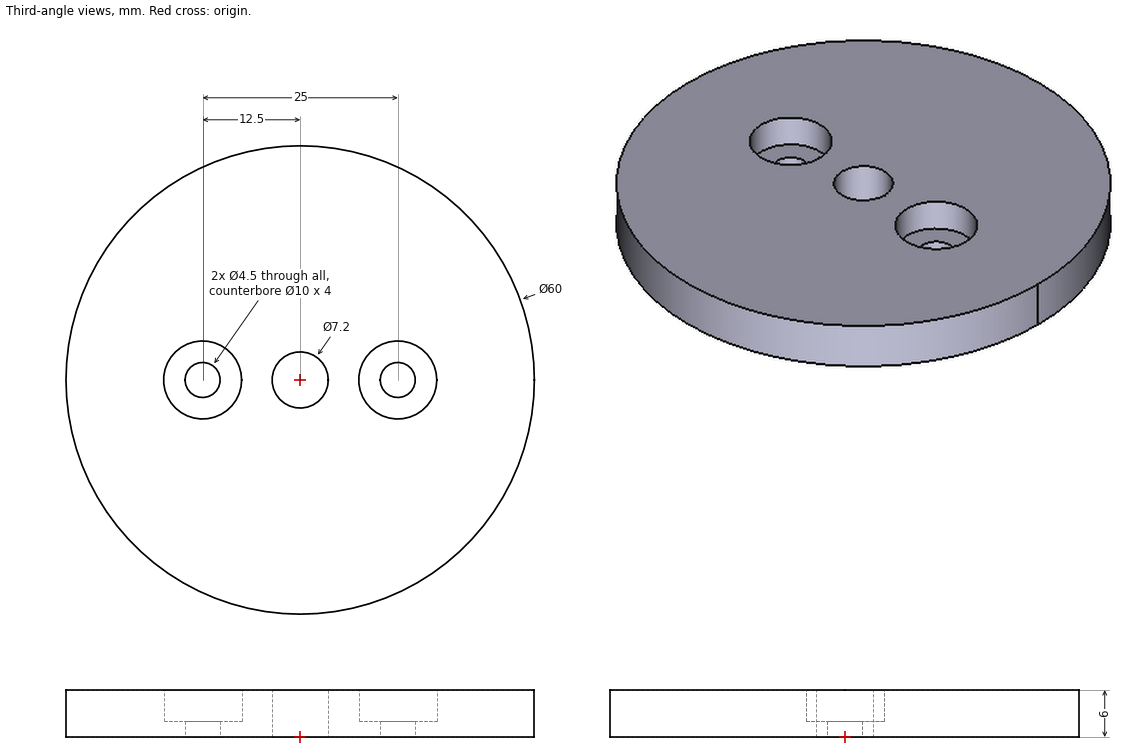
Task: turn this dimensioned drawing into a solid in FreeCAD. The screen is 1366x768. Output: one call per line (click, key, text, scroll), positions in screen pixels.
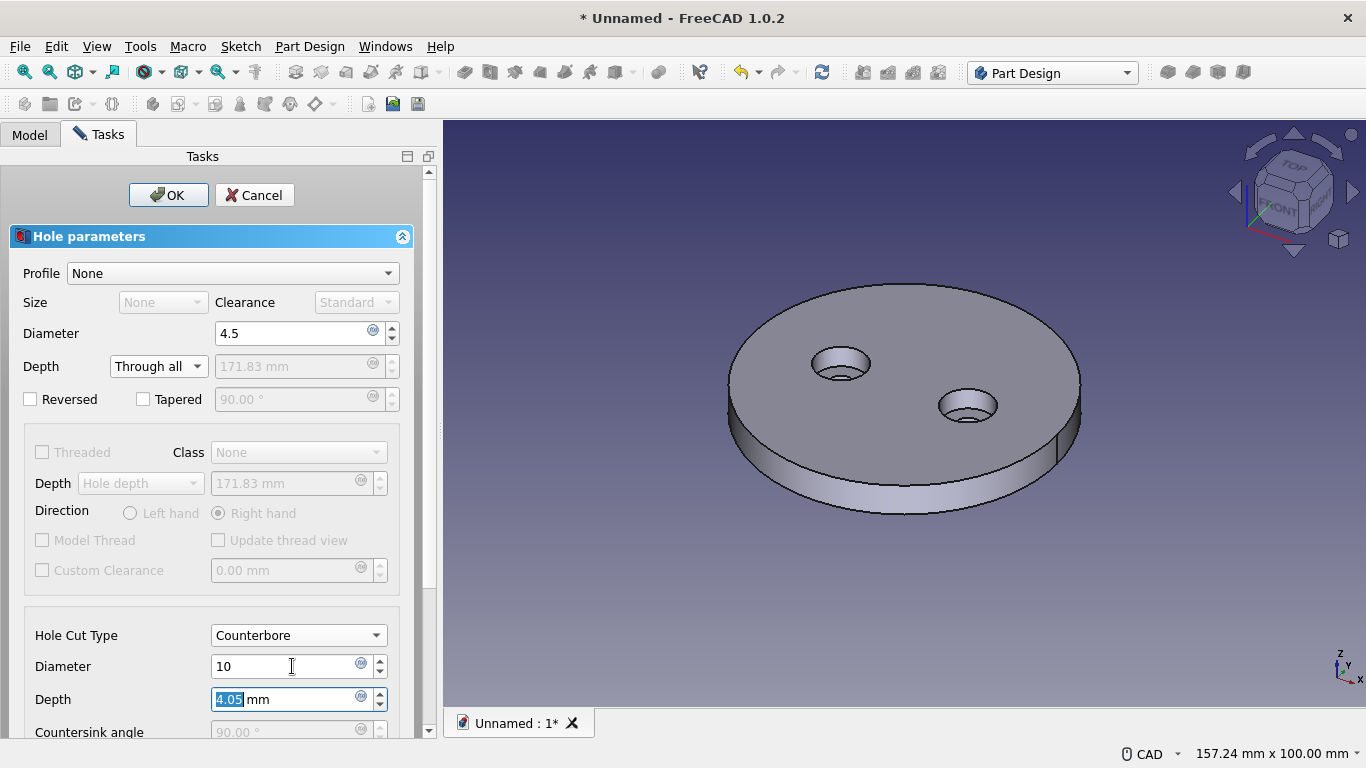
text(4)
key(Tab)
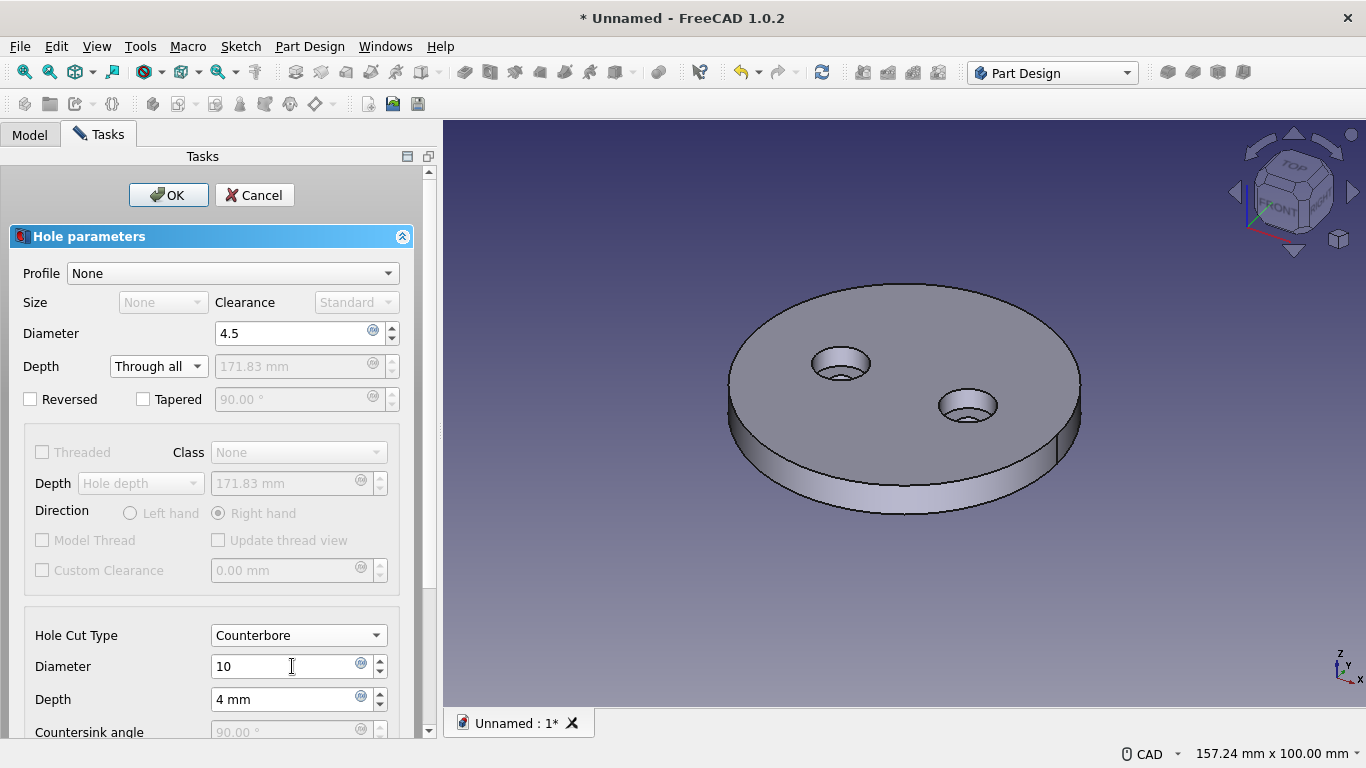
click(169, 195)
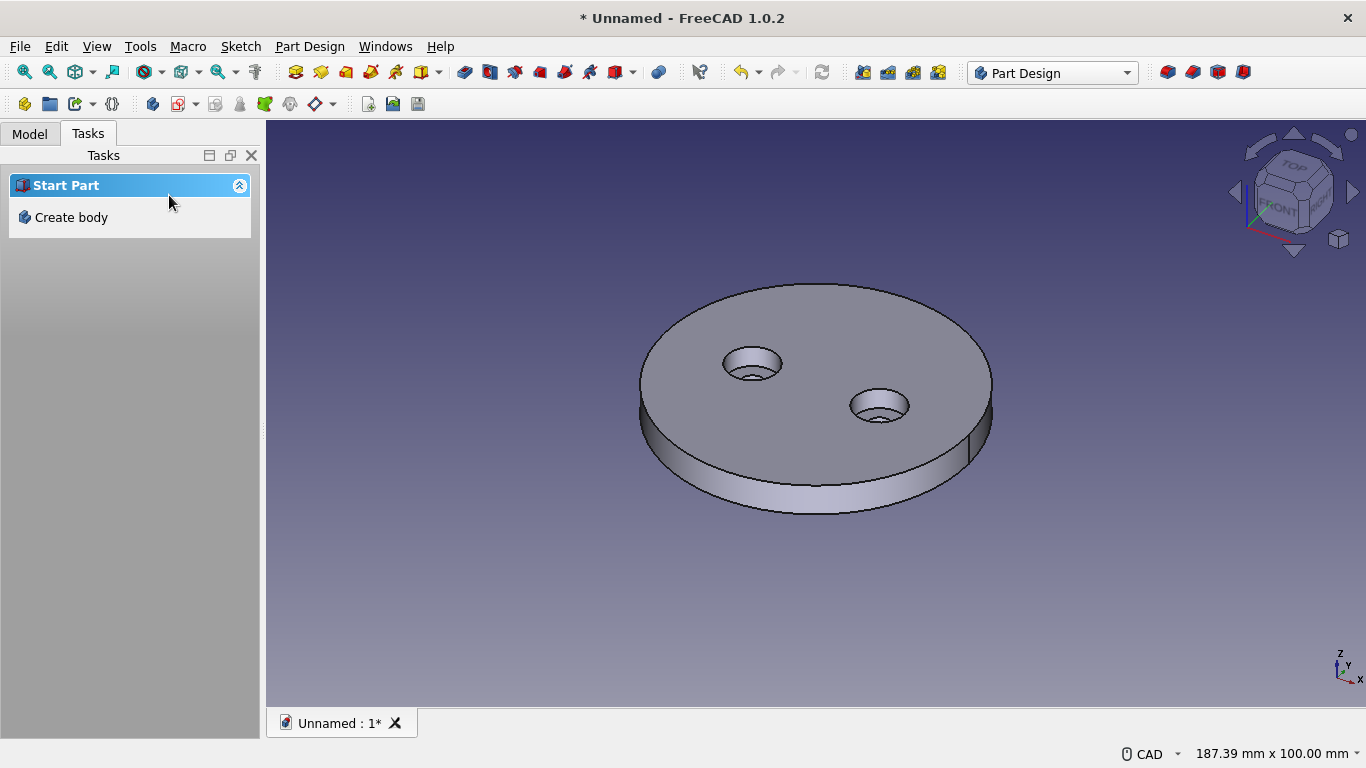
click(766, 434)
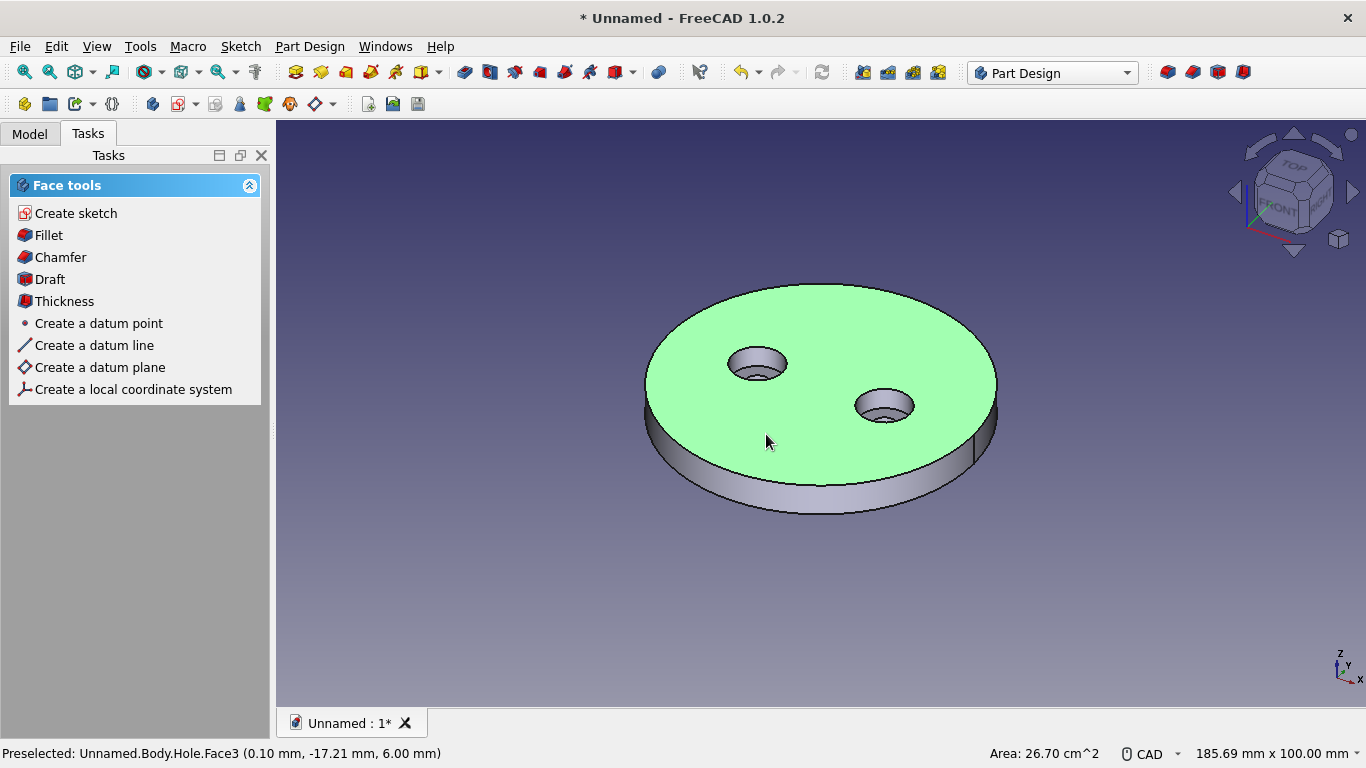
click(178, 104)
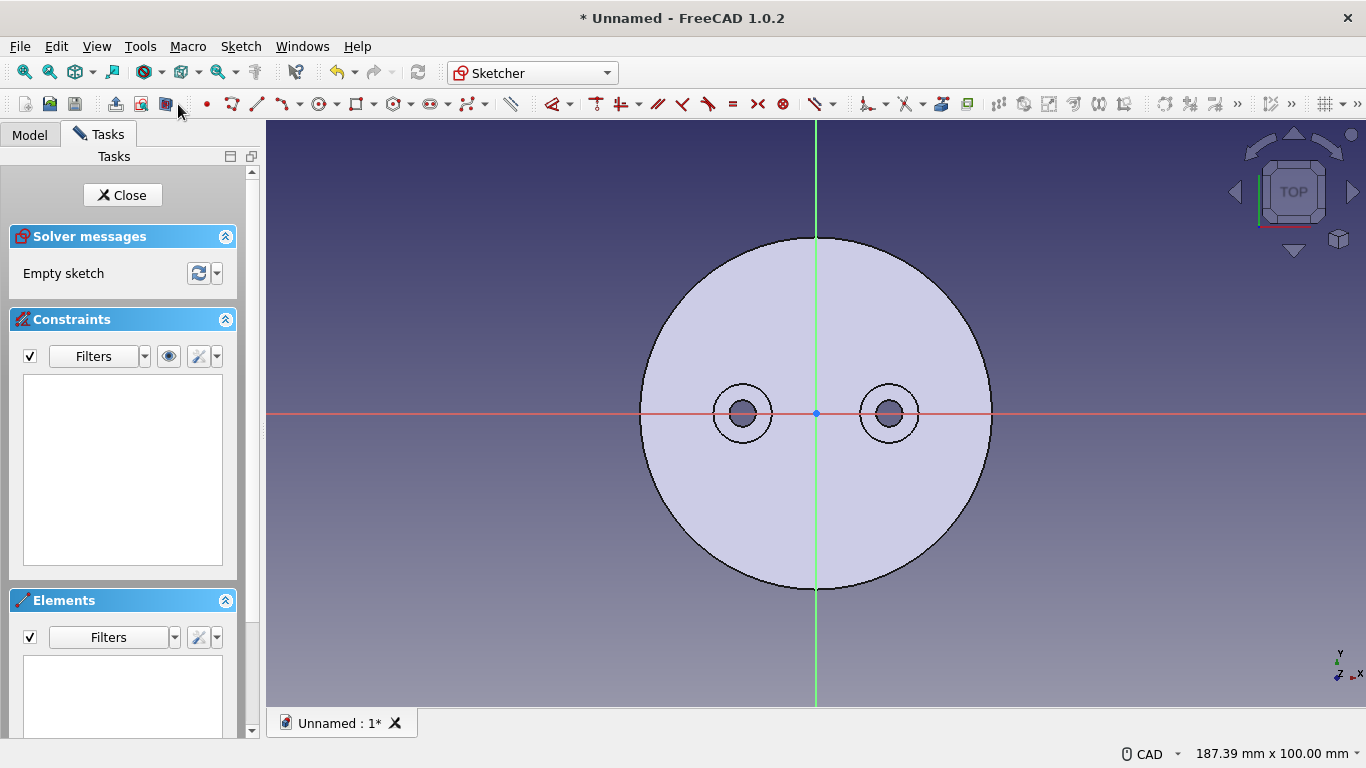
scroll(825, 414, up, 11)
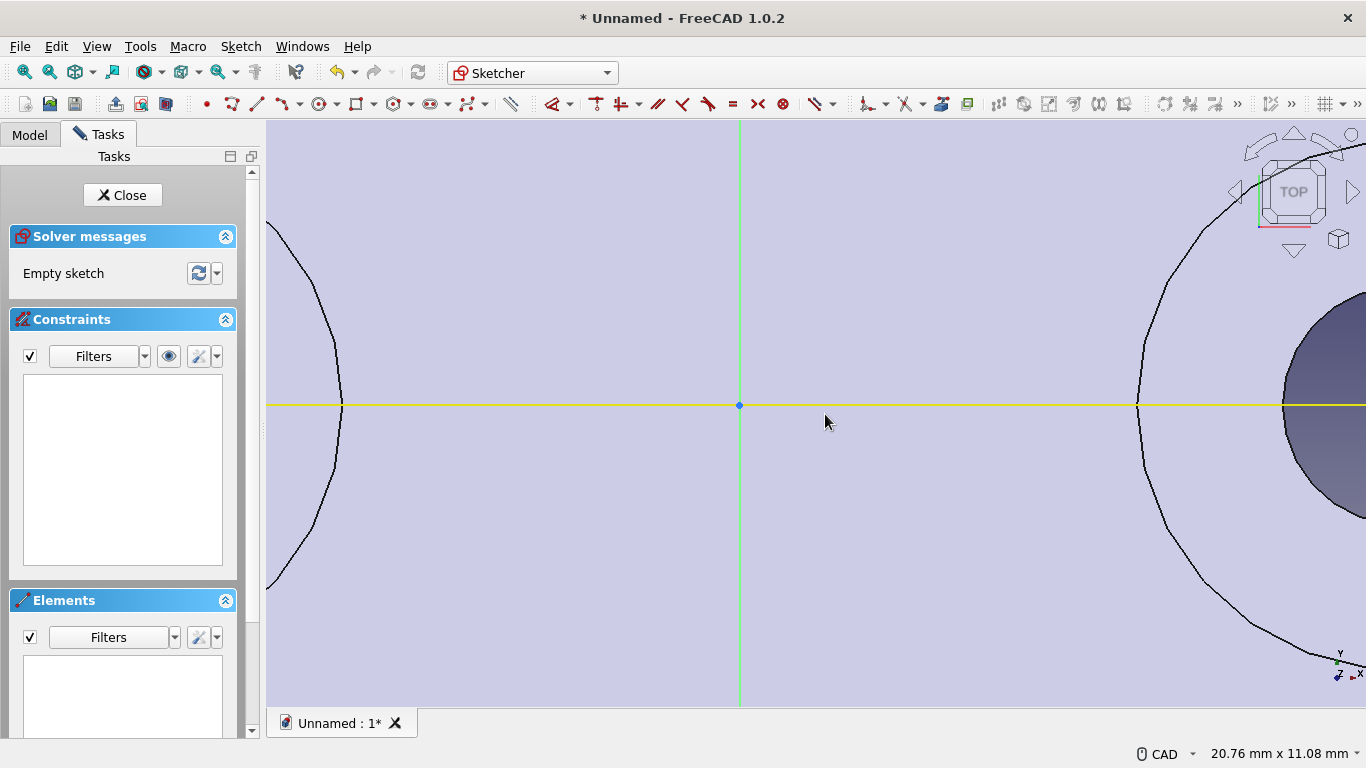
click(318, 104)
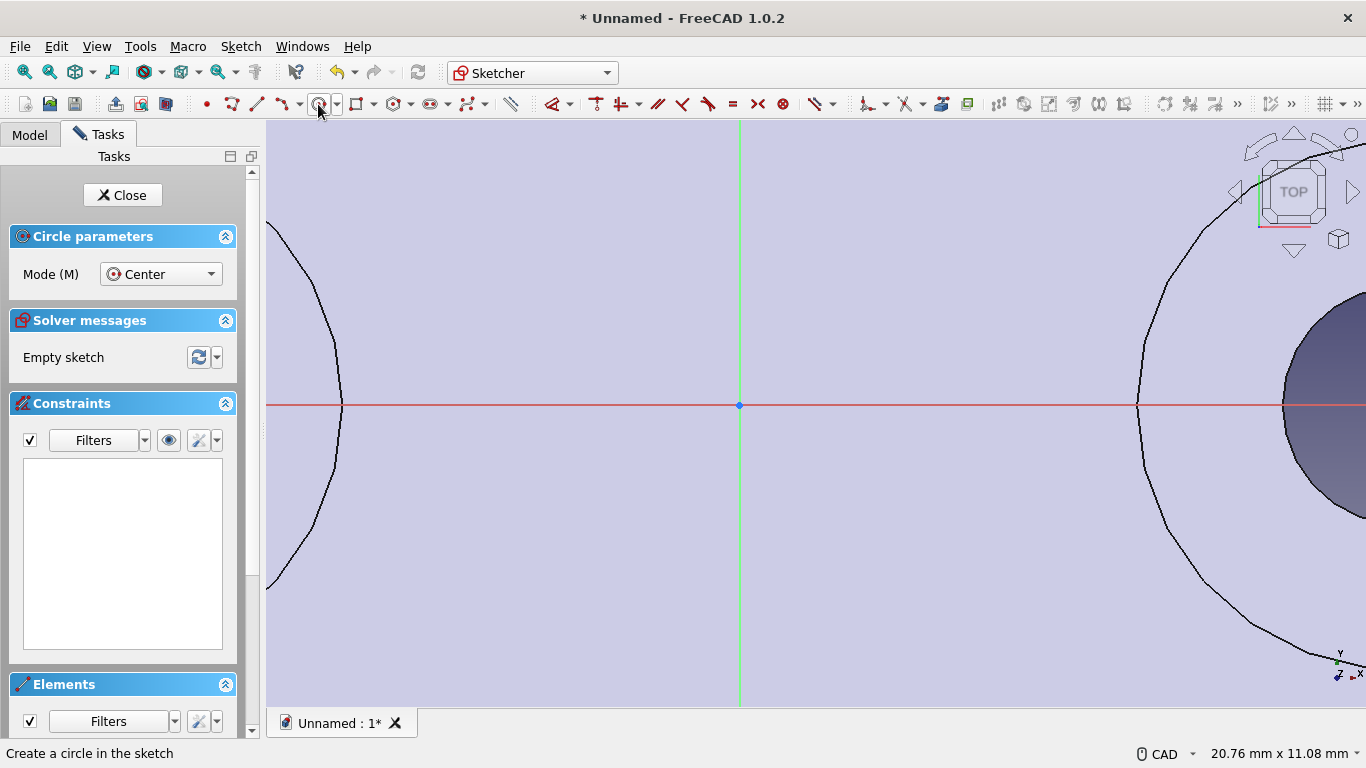
click(740, 405)
click(875, 271)
key(Escape)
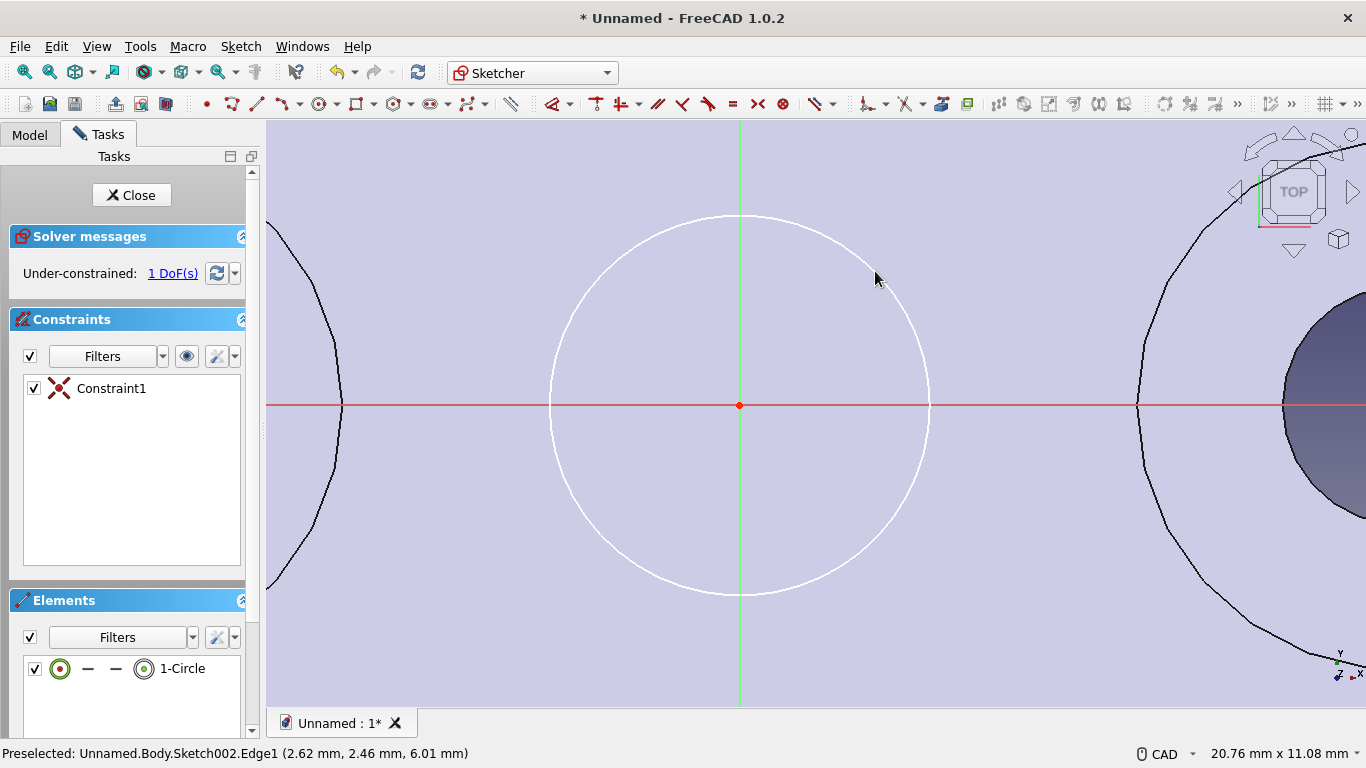
click(552, 104)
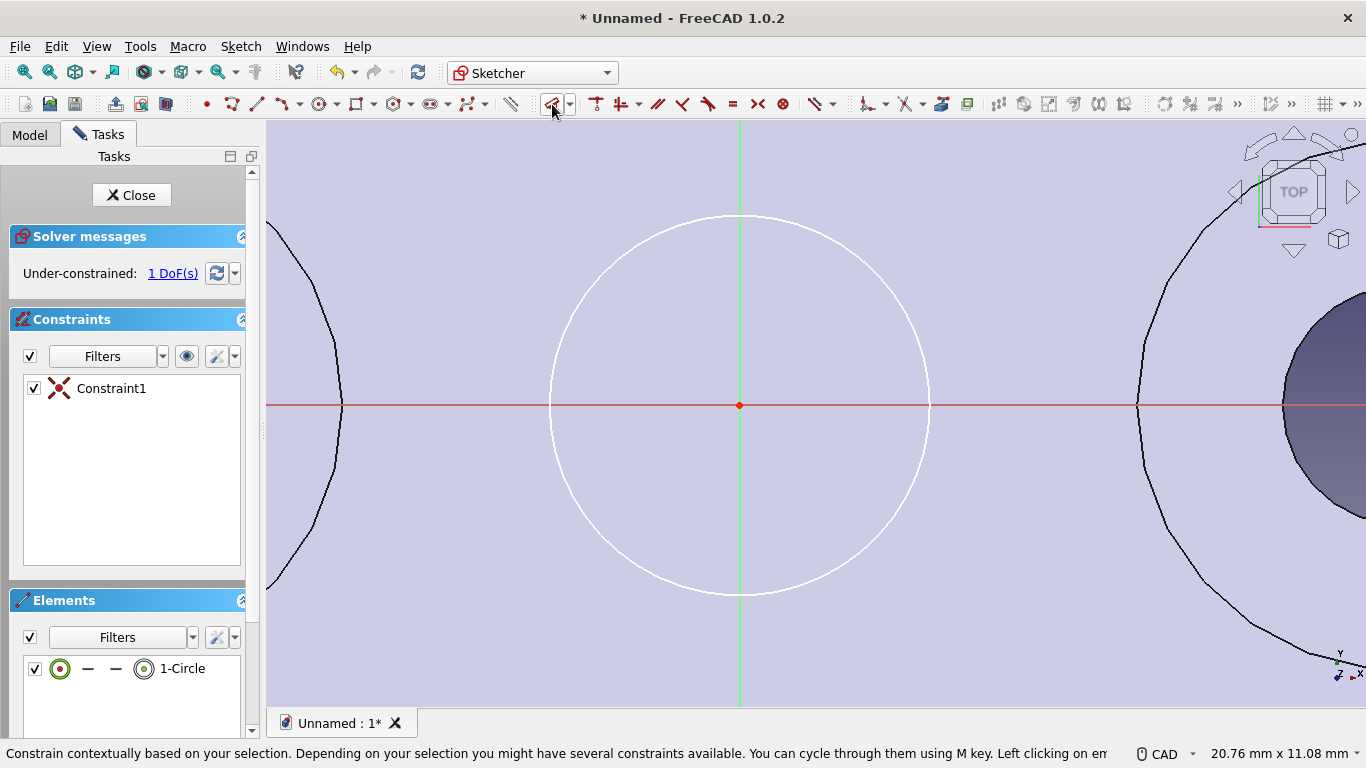
click(874, 271)
click(897, 248)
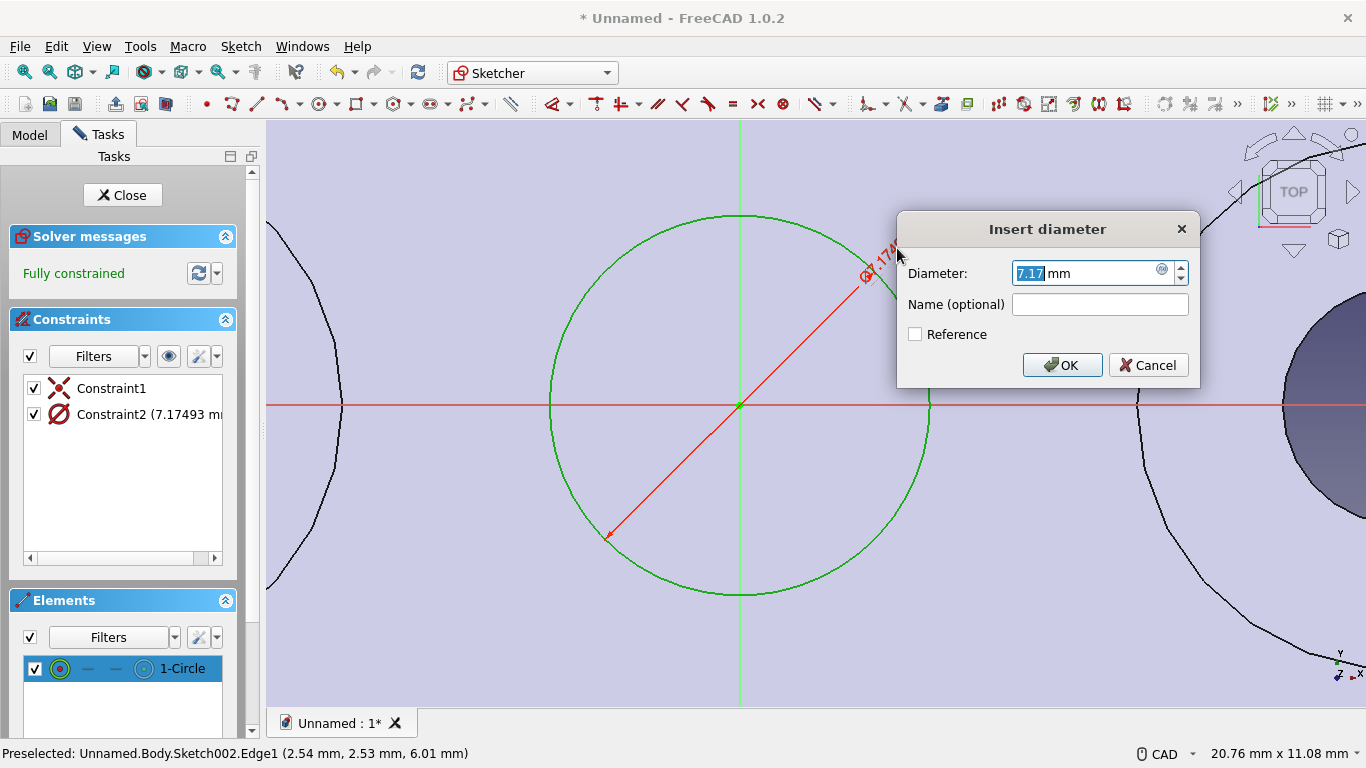
text(7.2)
key(Return)
key(Escape)